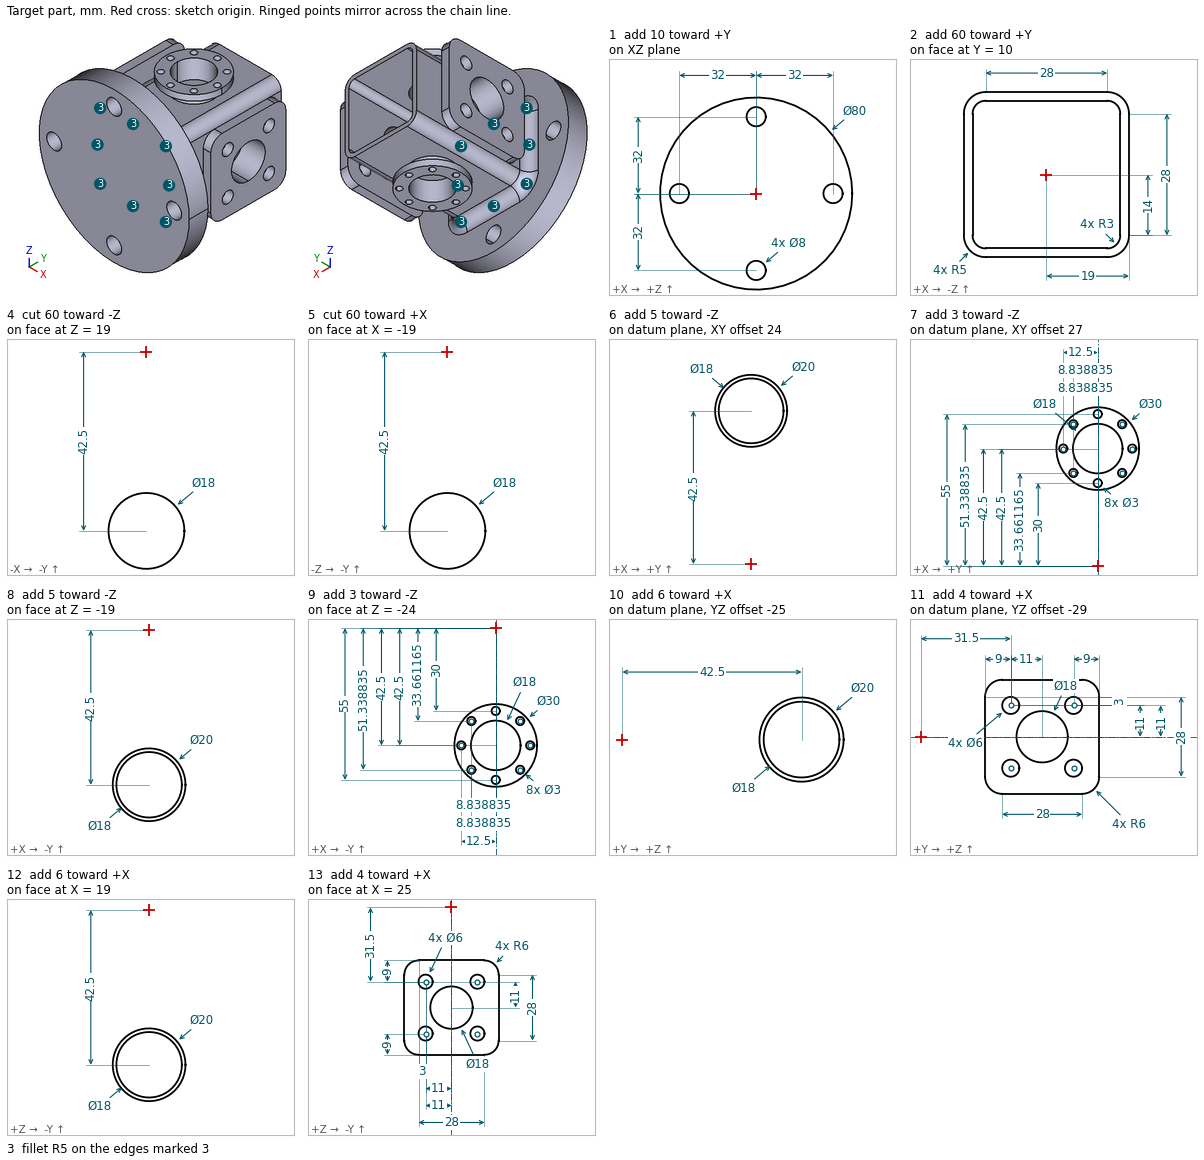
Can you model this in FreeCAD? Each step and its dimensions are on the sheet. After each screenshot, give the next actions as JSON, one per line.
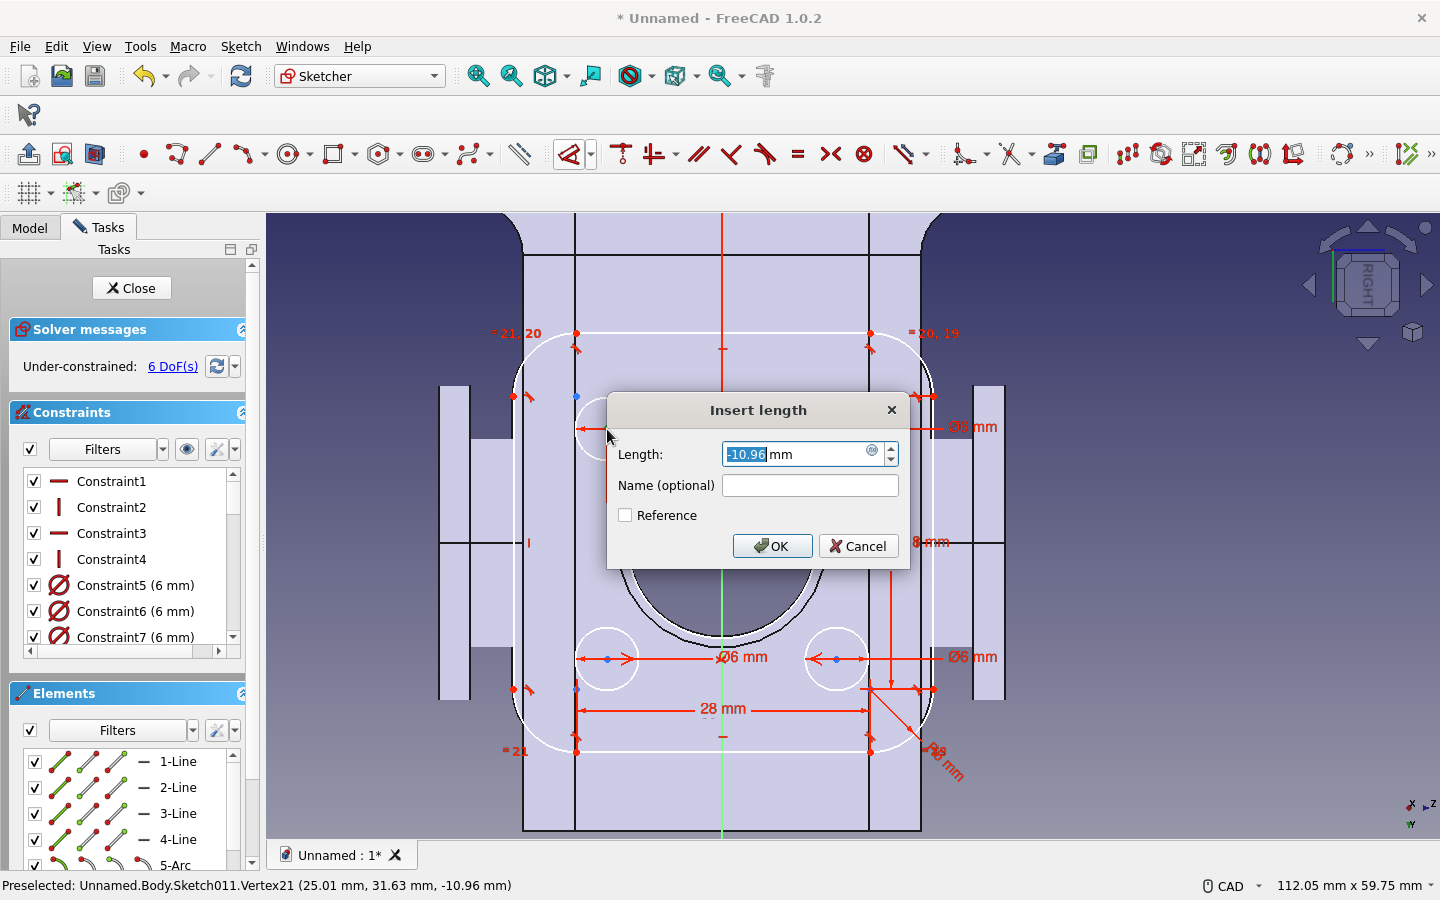
{"action": "type", "text": "-11"}
{"action": "key", "text": "Return"}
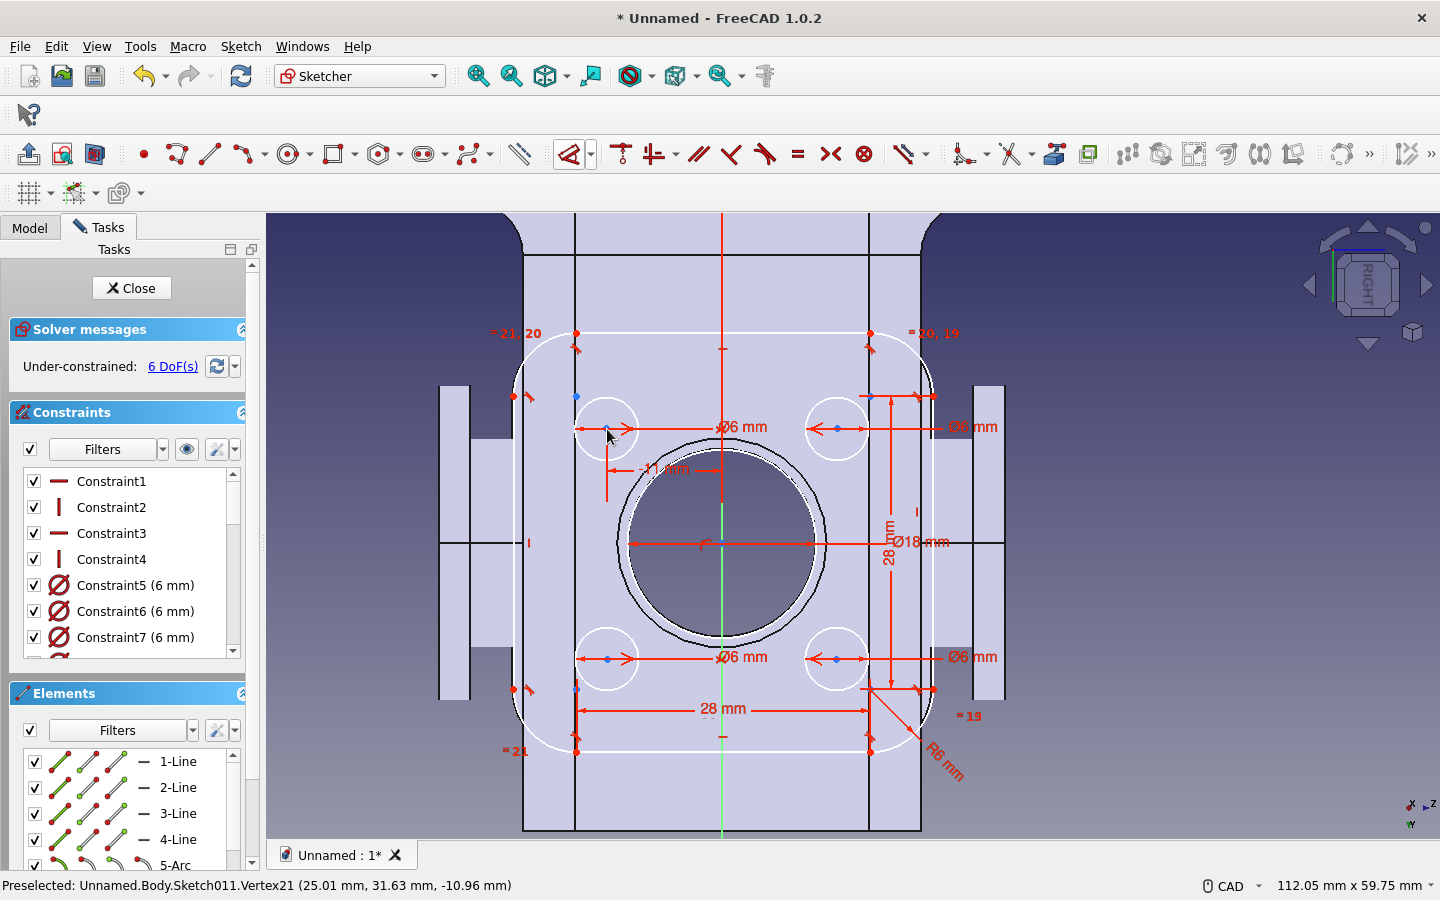
{"action": "left_click", "coordinate": [607, 659]}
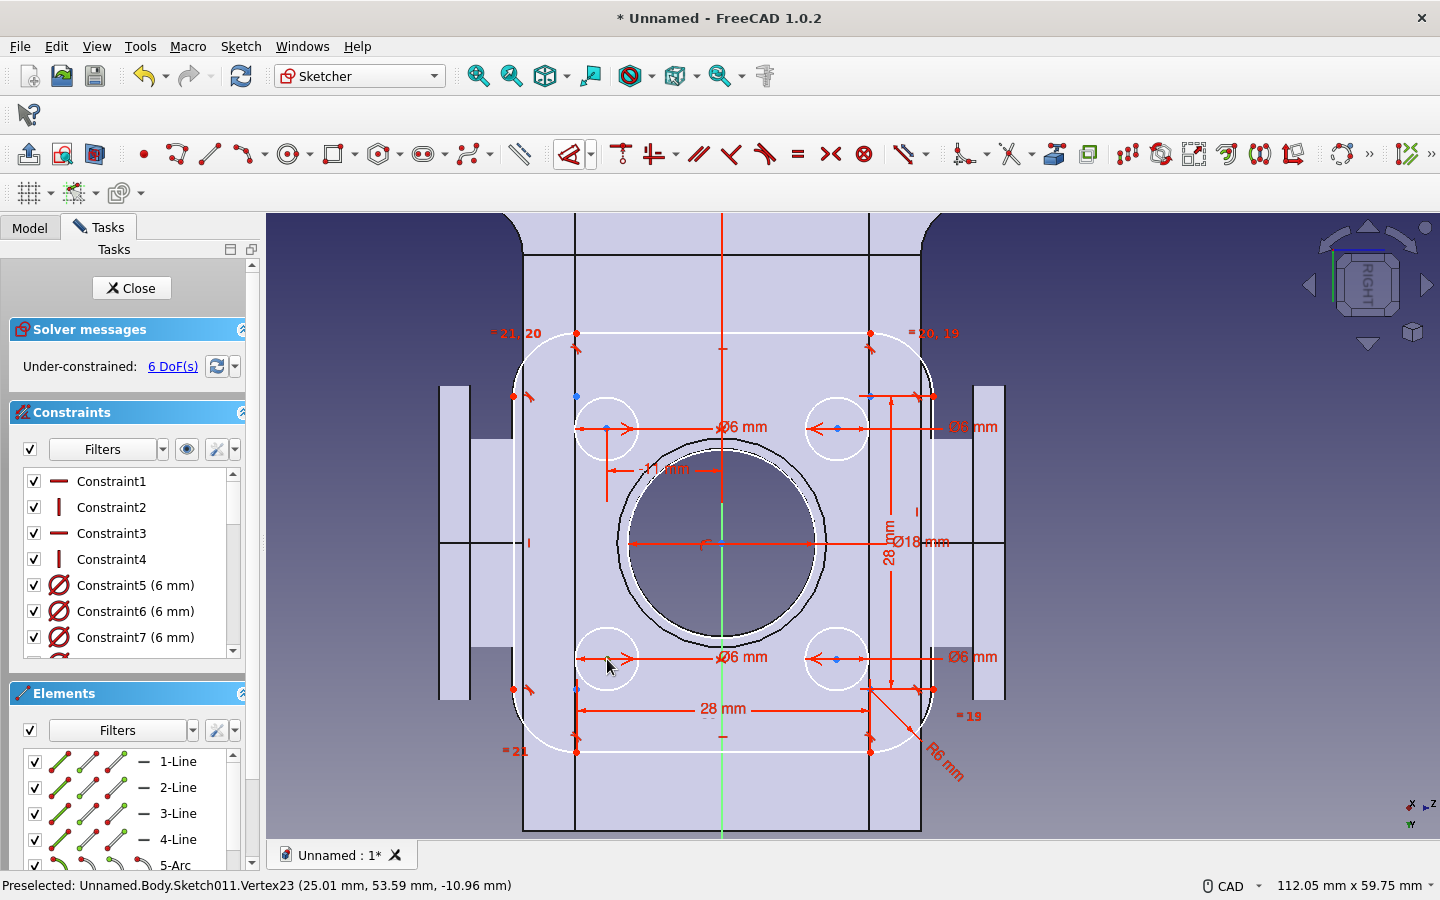
{"action": "key", "text": "l"}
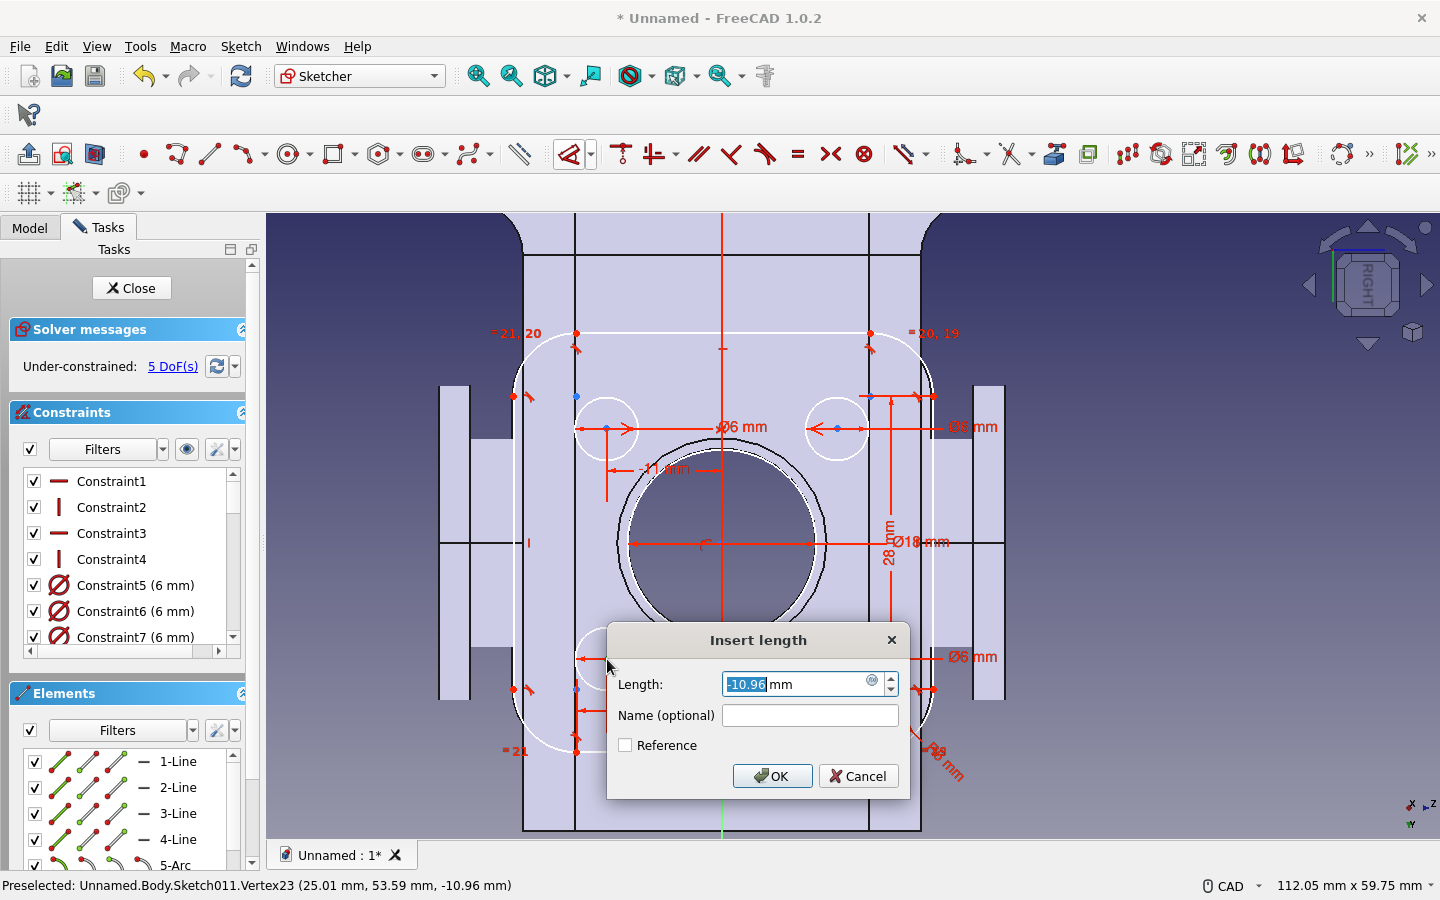
{"action": "type", "text": "-11"}
{"action": "key", "text": "Return"}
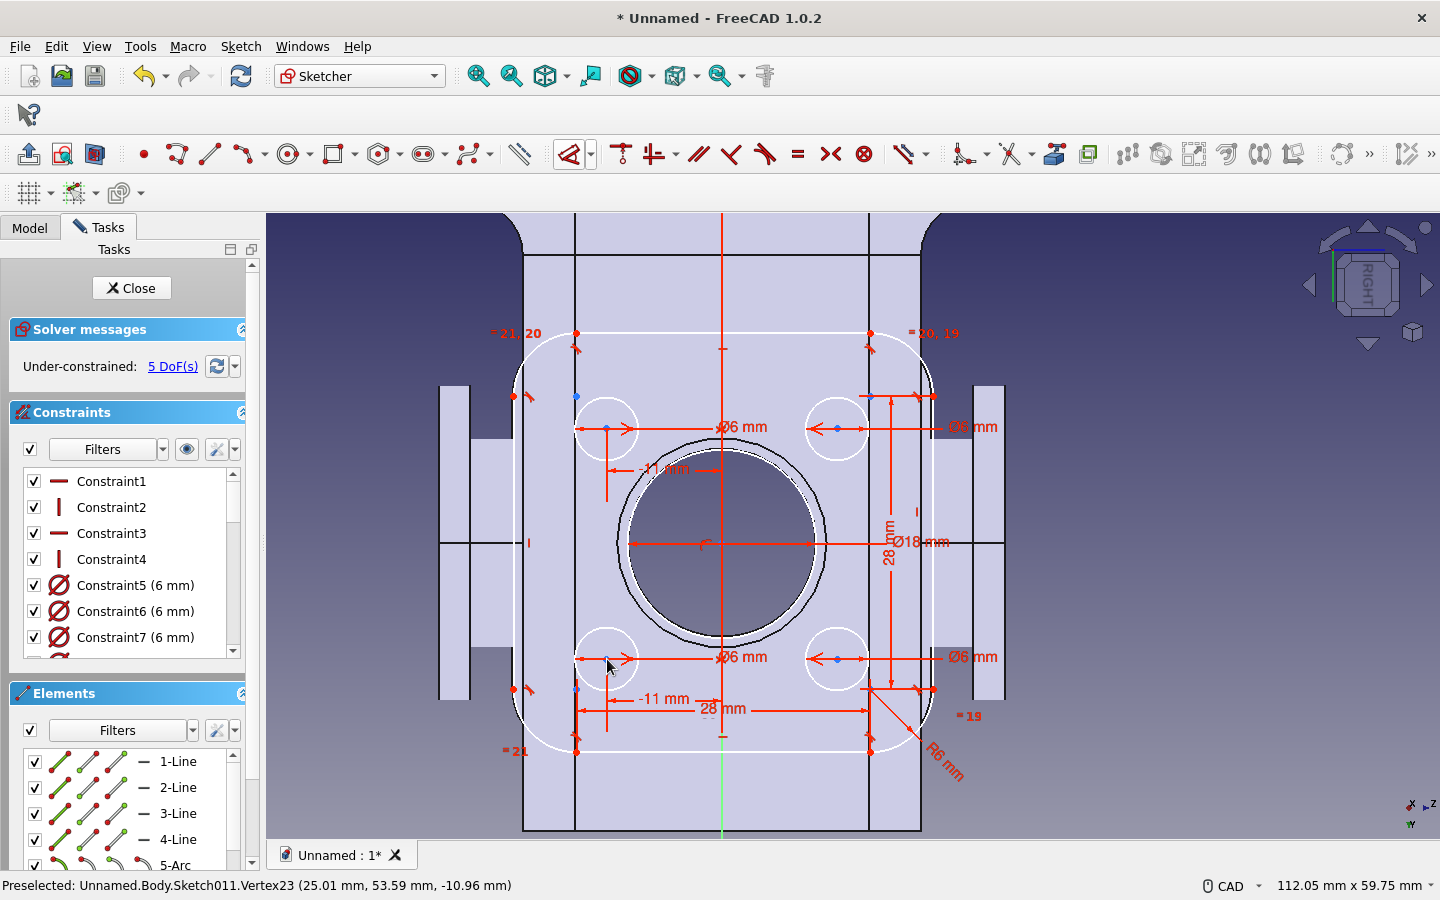
{"action": "scroll", "coordinate": [577, 333], "scroll_direction": "up", "scroll_amount": 2}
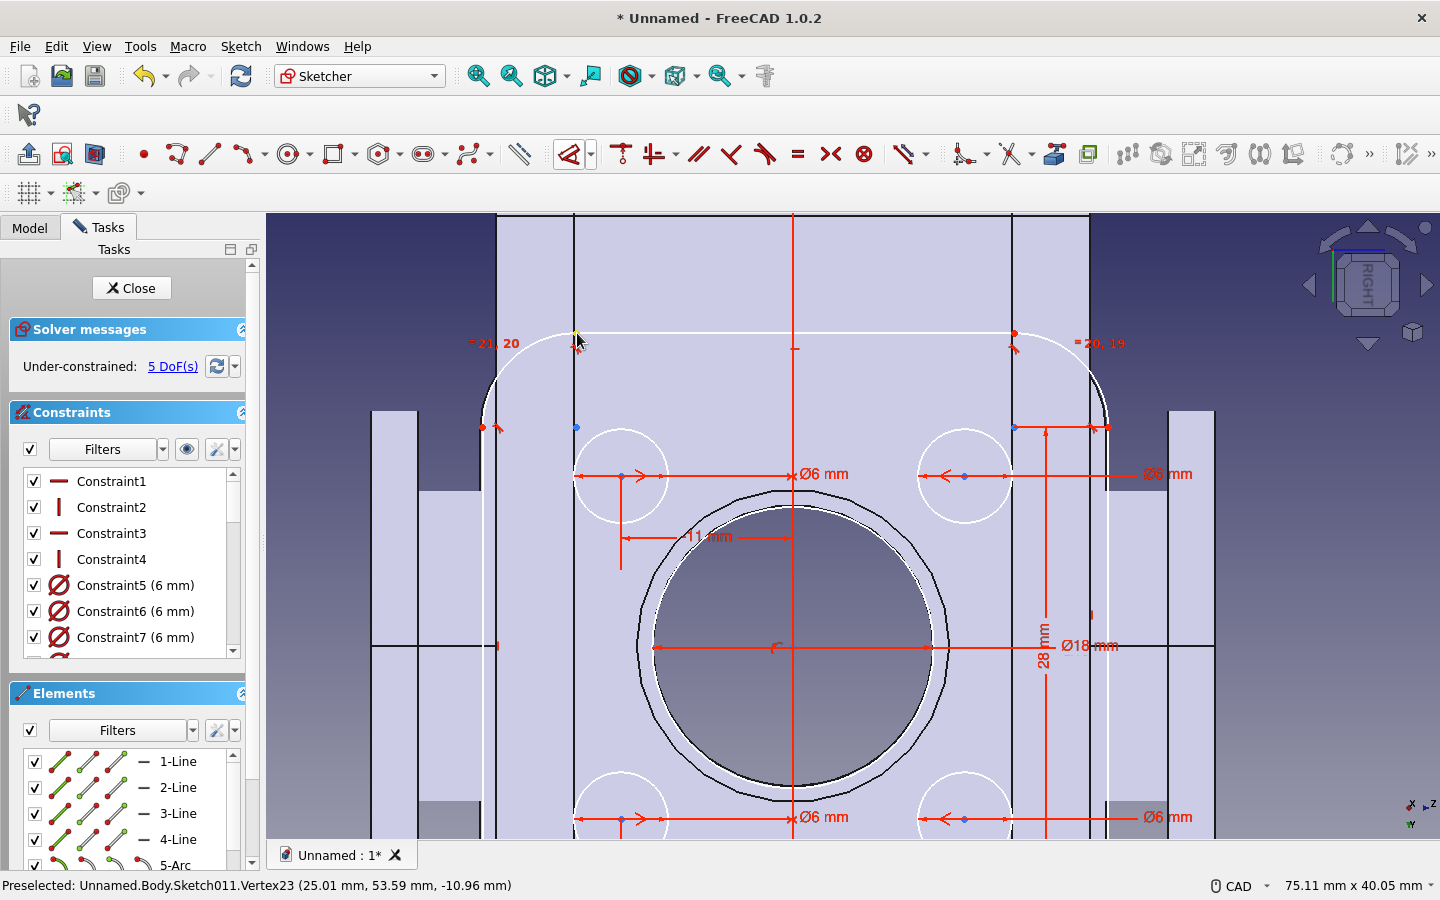
{"action": "left_click", "coordinate": [577, 333]}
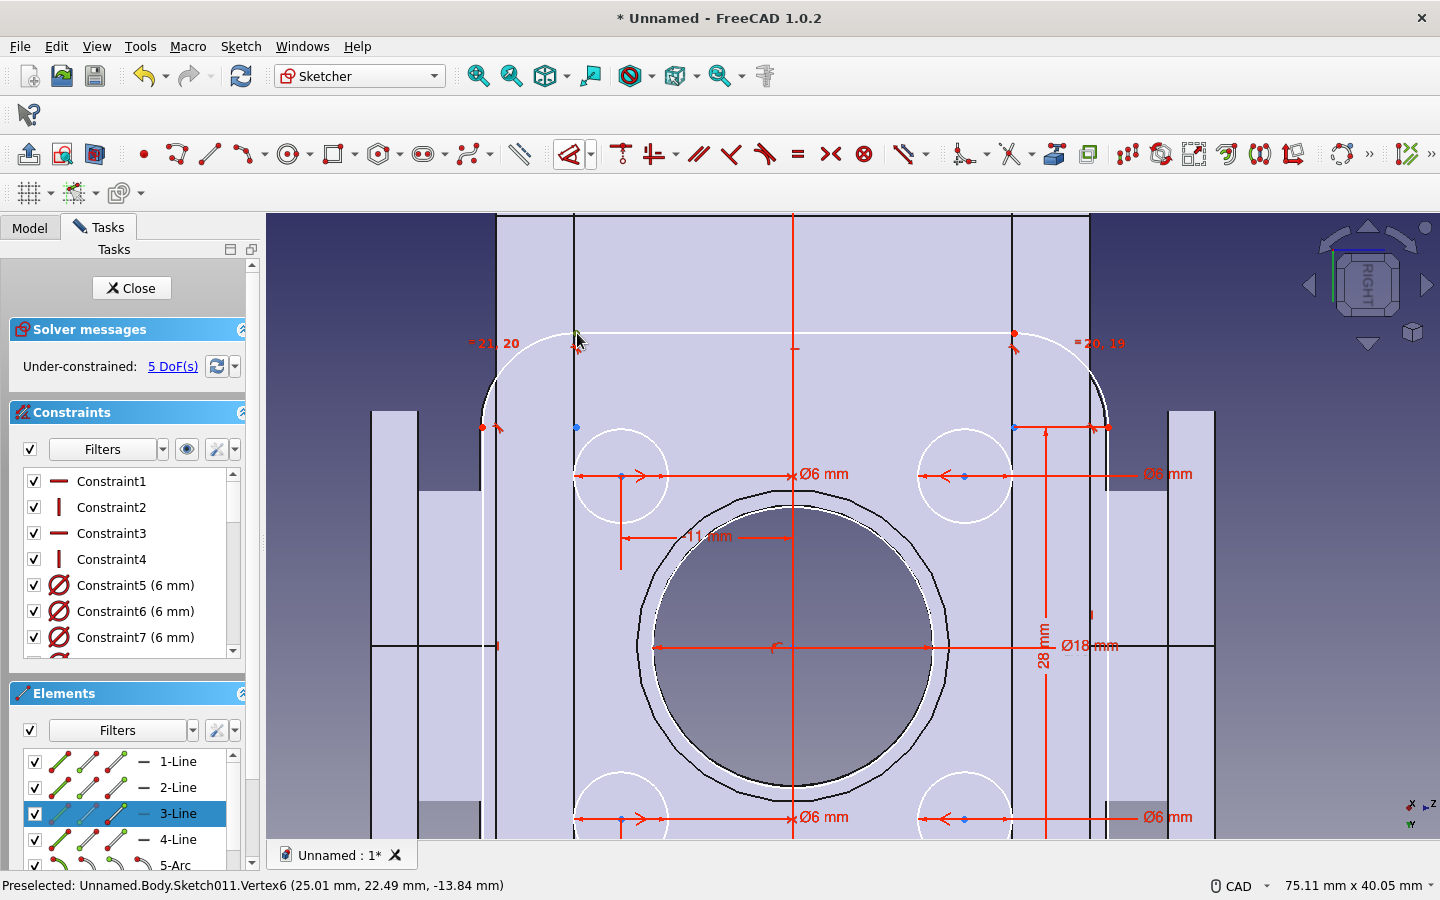
{"action": "left_click", "coordinate": [621, 476]}